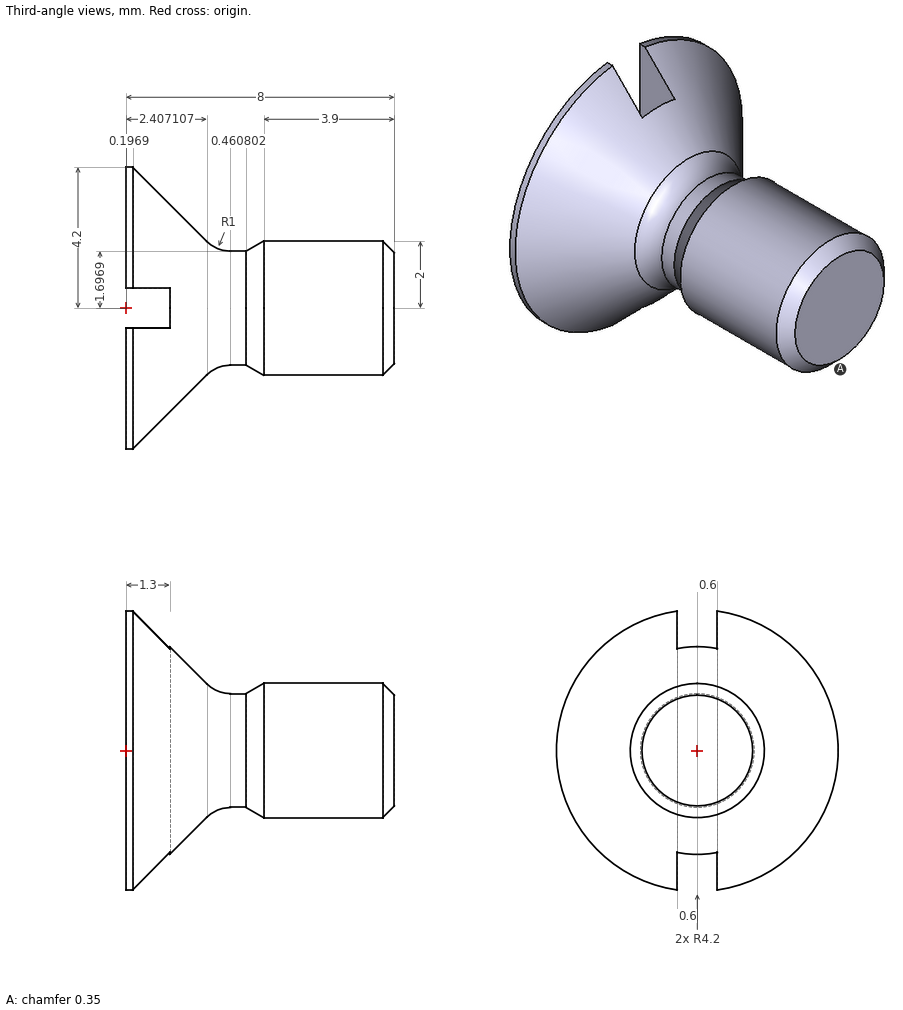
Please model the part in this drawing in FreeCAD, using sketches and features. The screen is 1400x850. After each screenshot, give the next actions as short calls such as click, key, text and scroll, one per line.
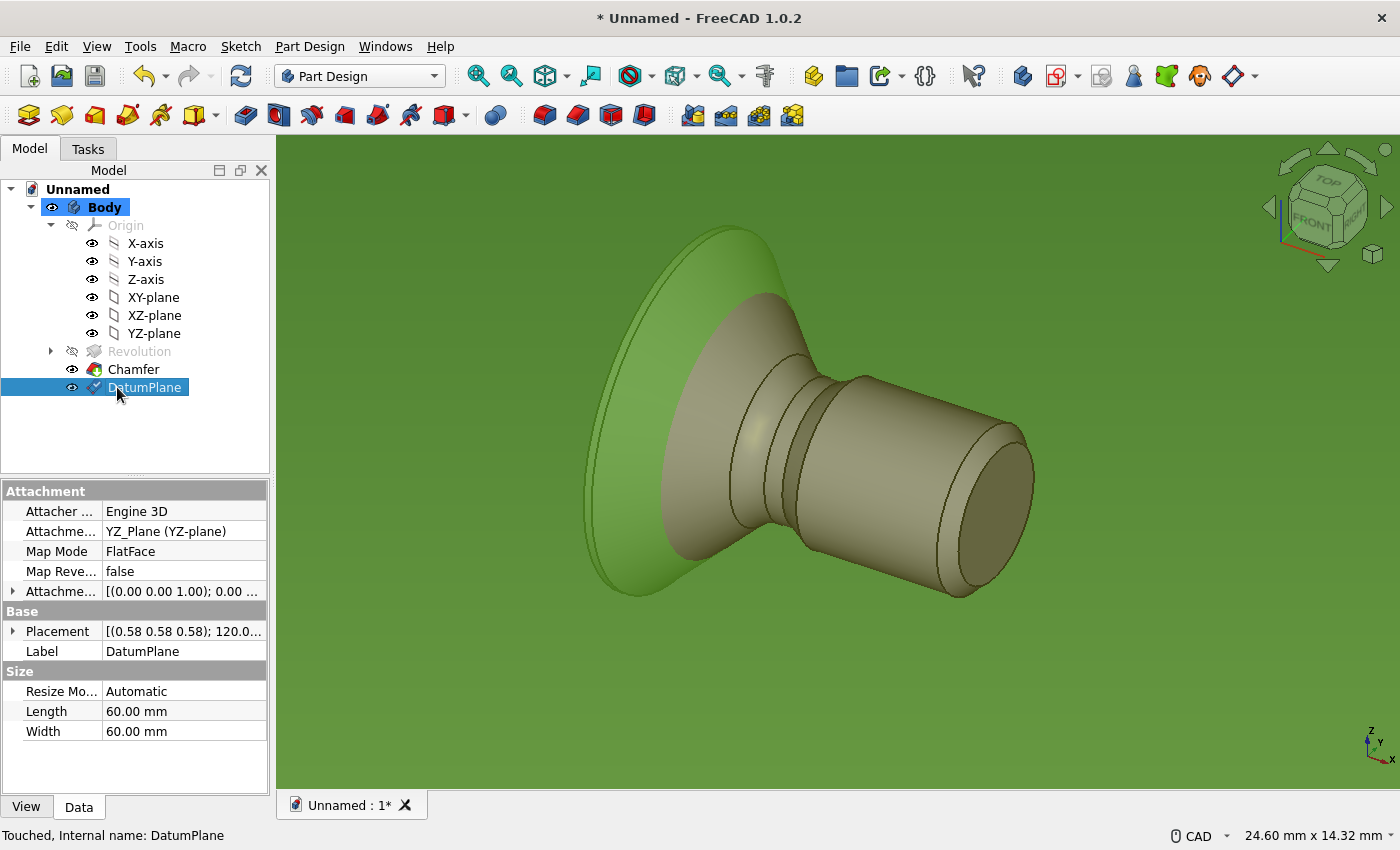
click(1056, 76)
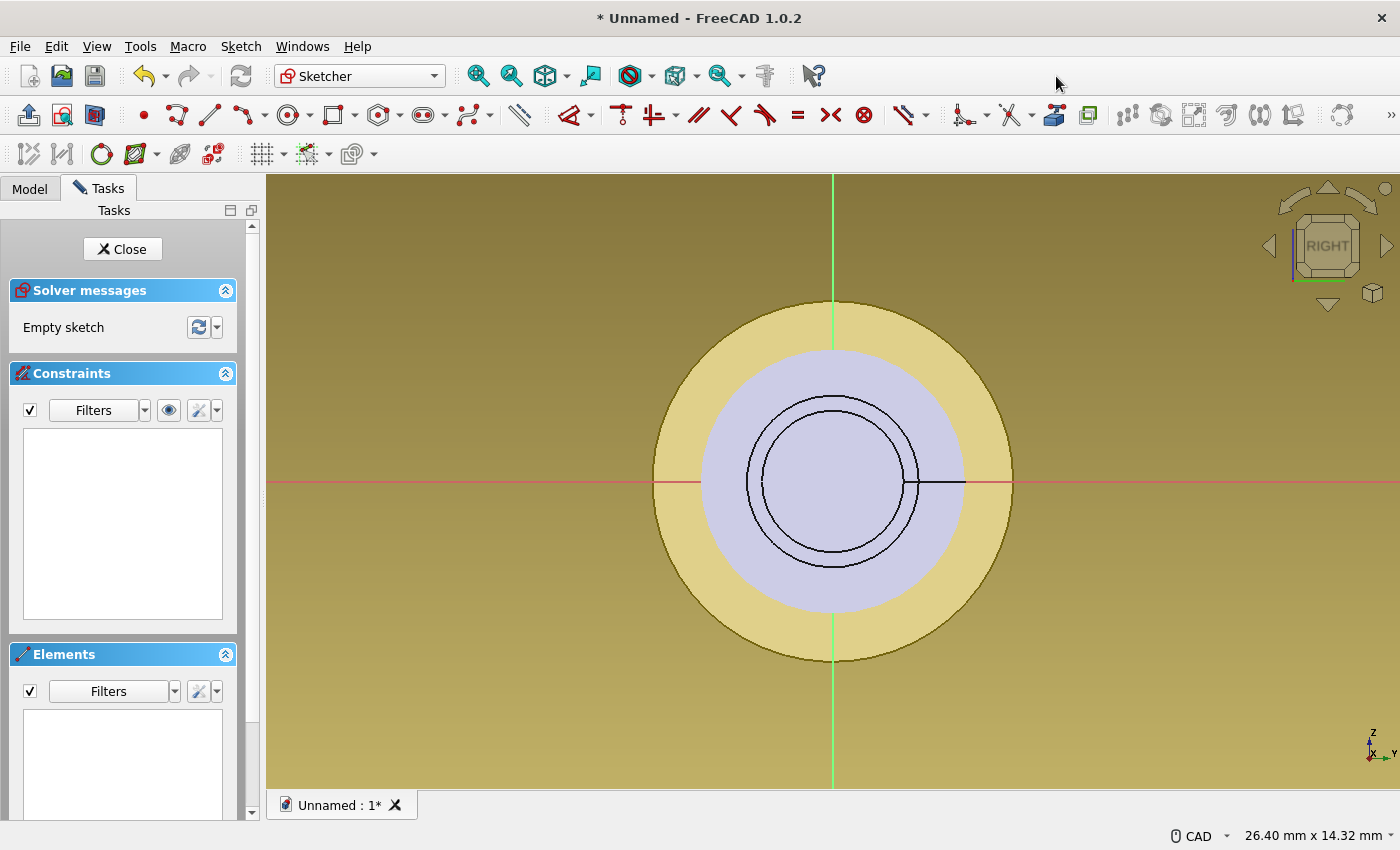
key(q)
key(s)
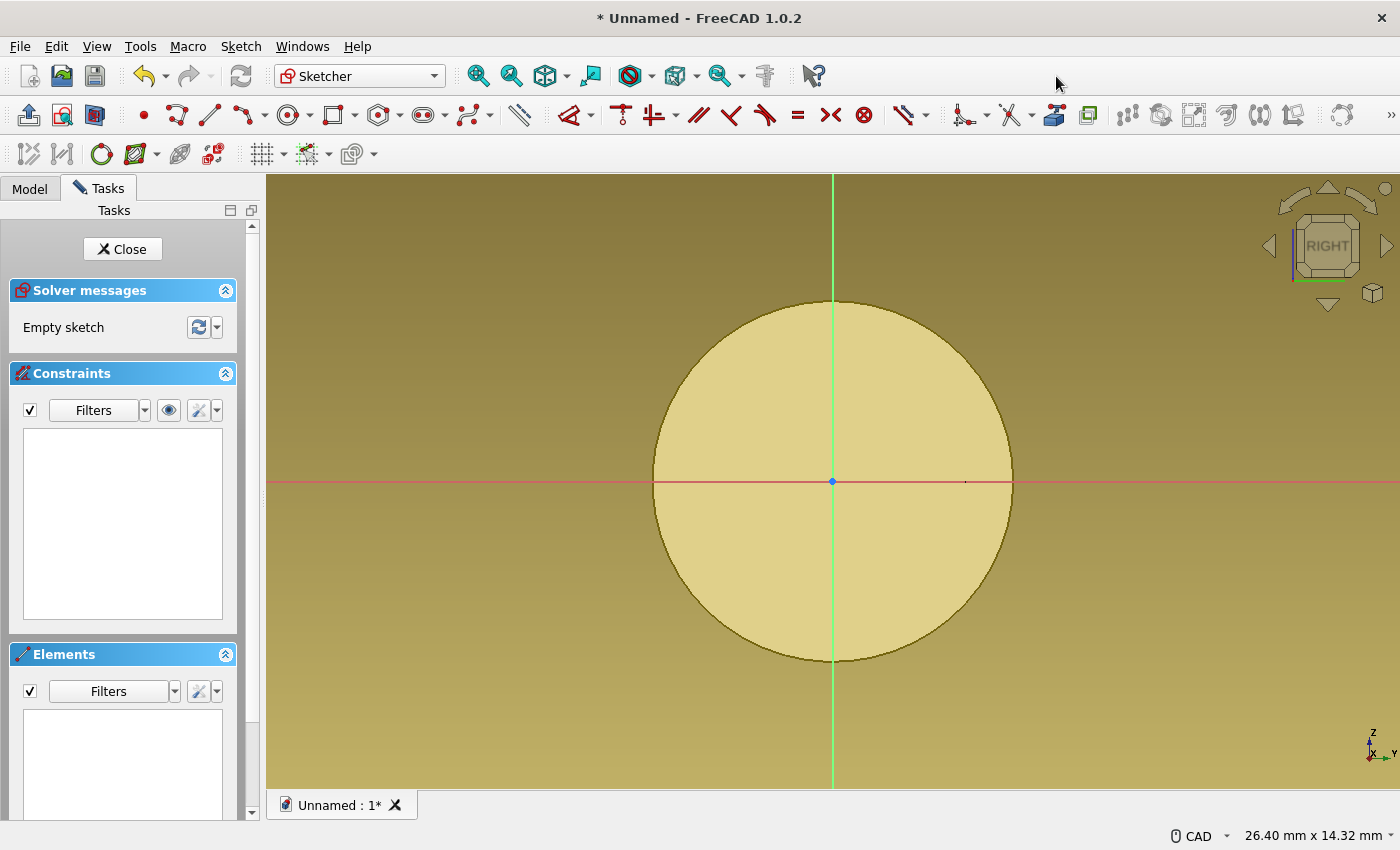
click(210, 116)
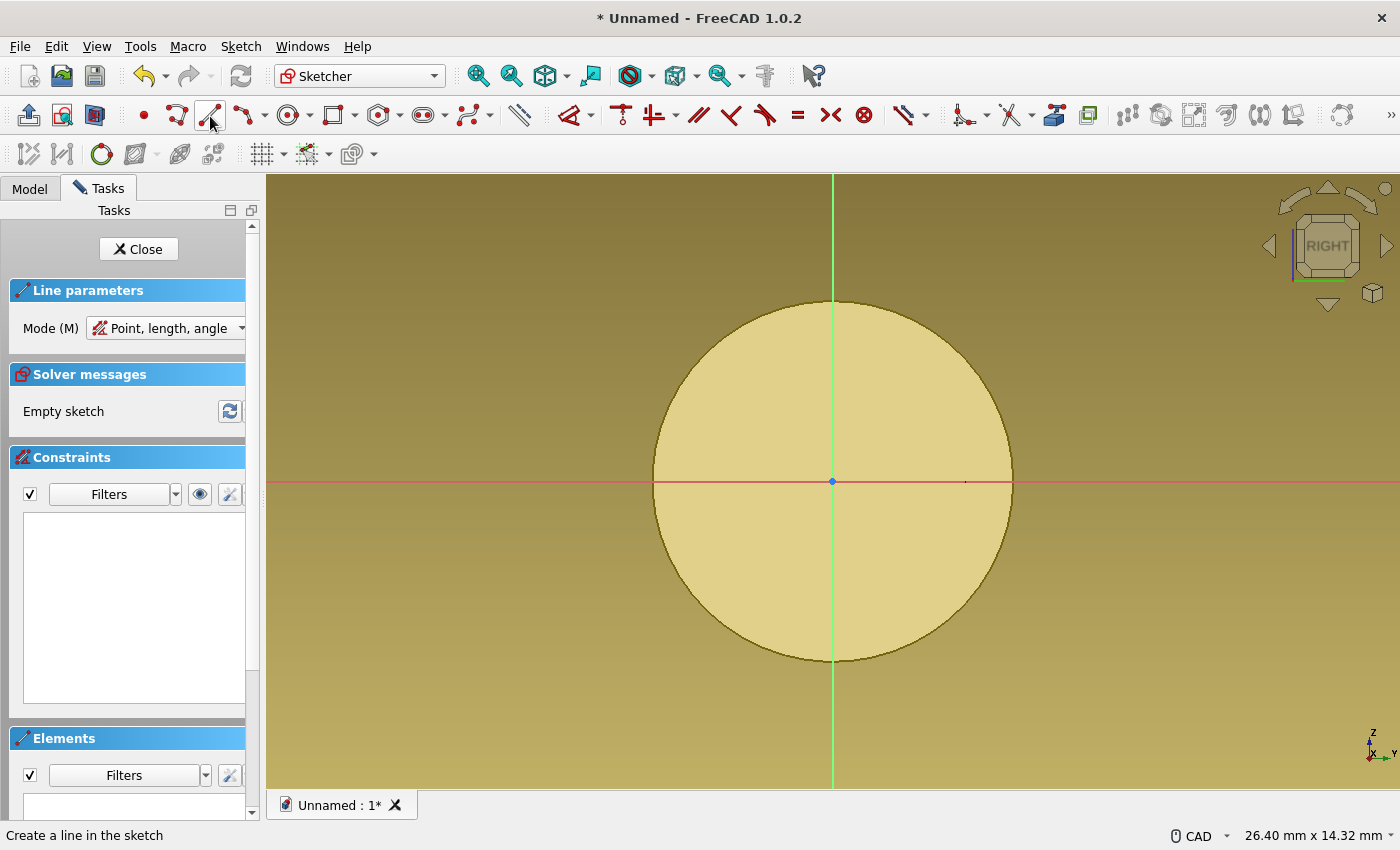
click(859, 303)
click(859, 660)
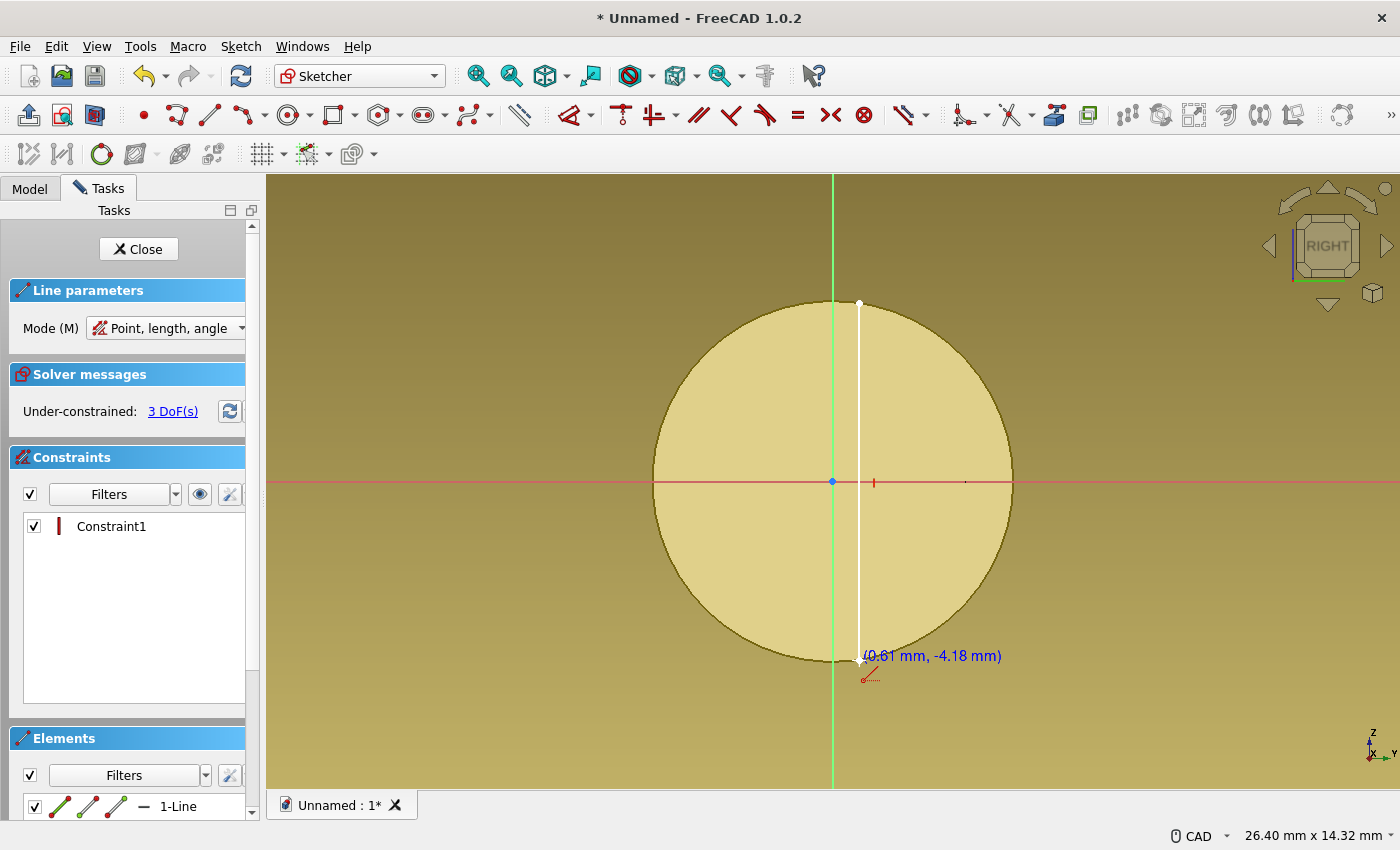
click(807, 660)
click(807, 303)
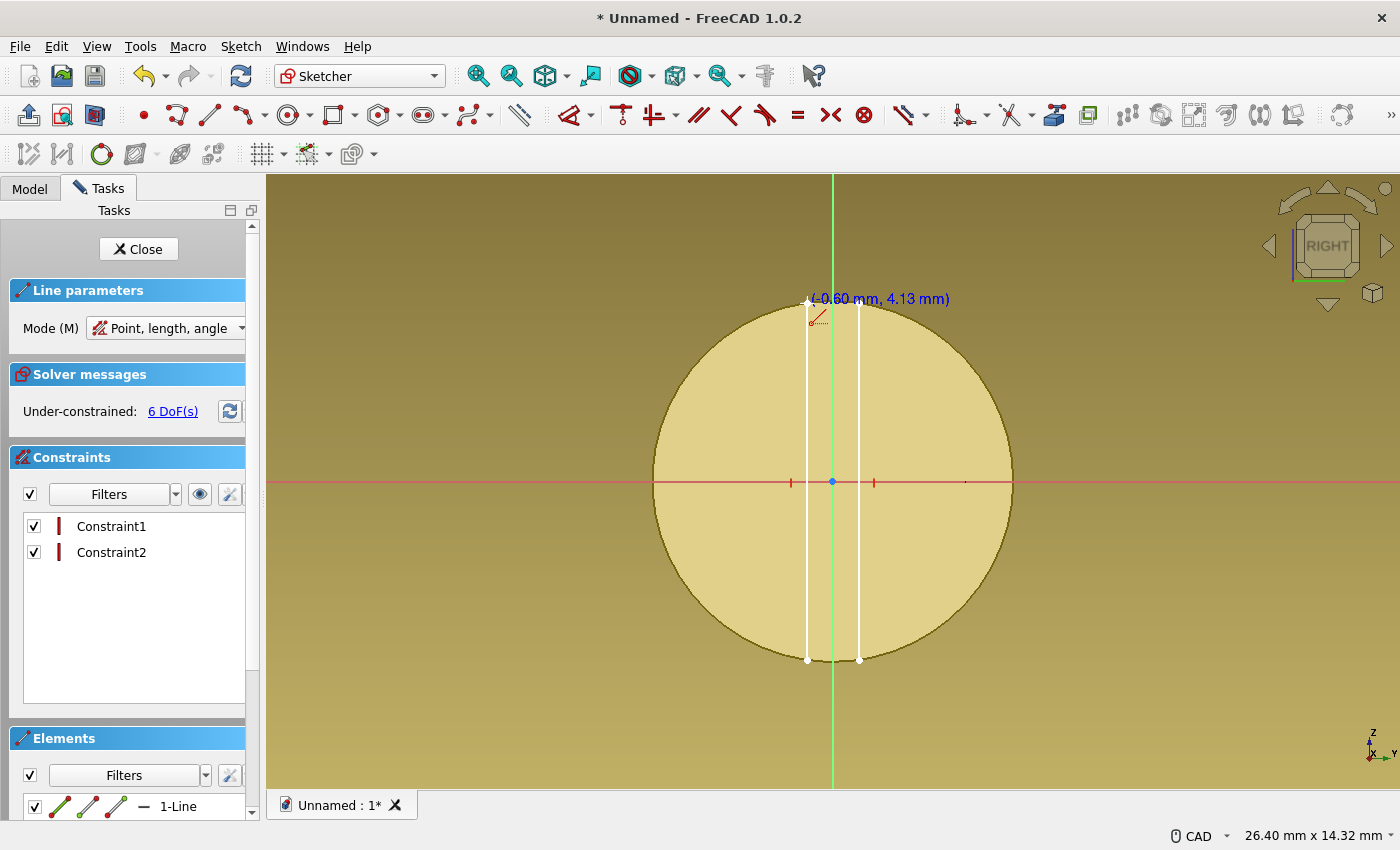
key(g)
key(3)
key(a)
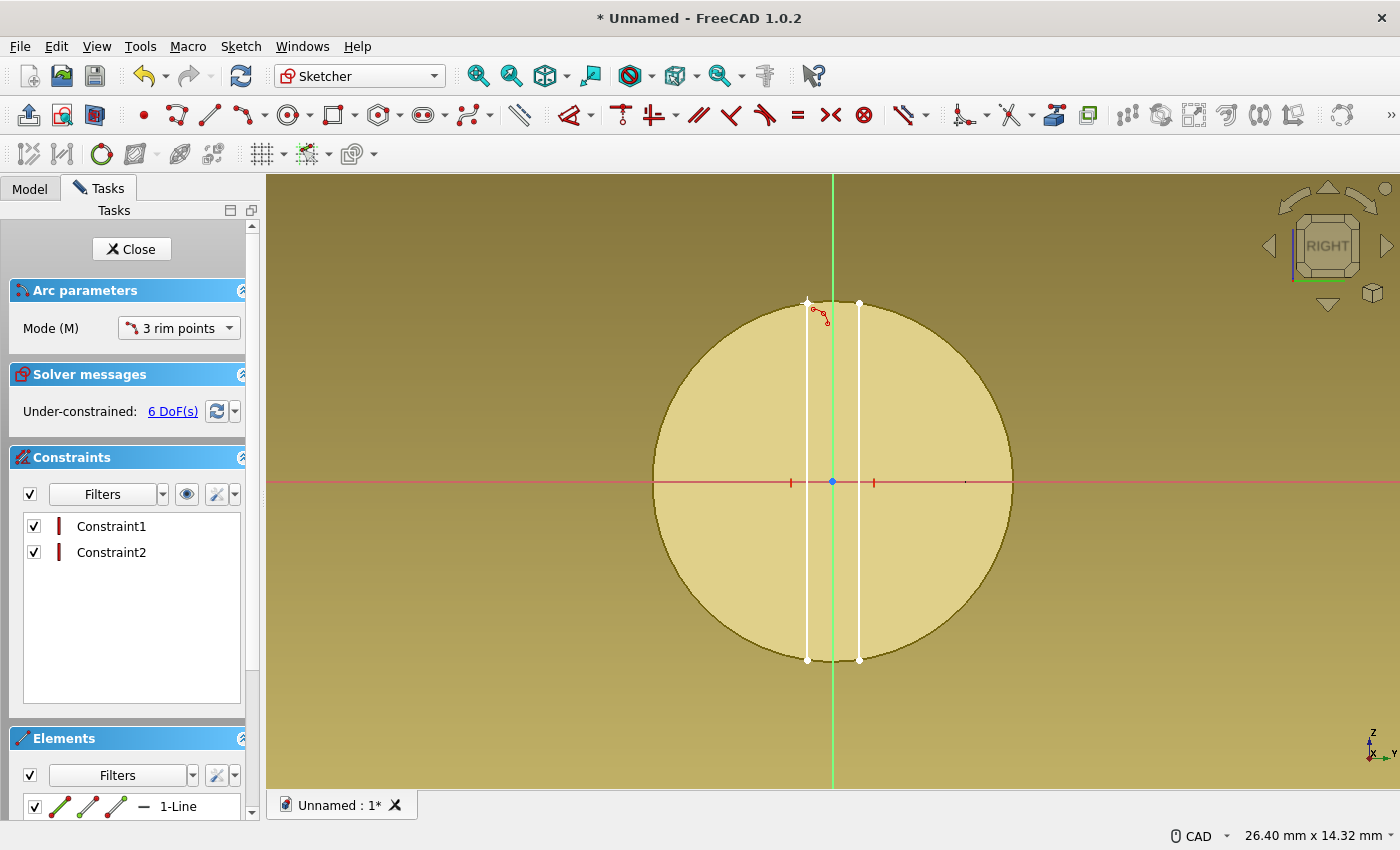
click(859, 661)
click(807, 661)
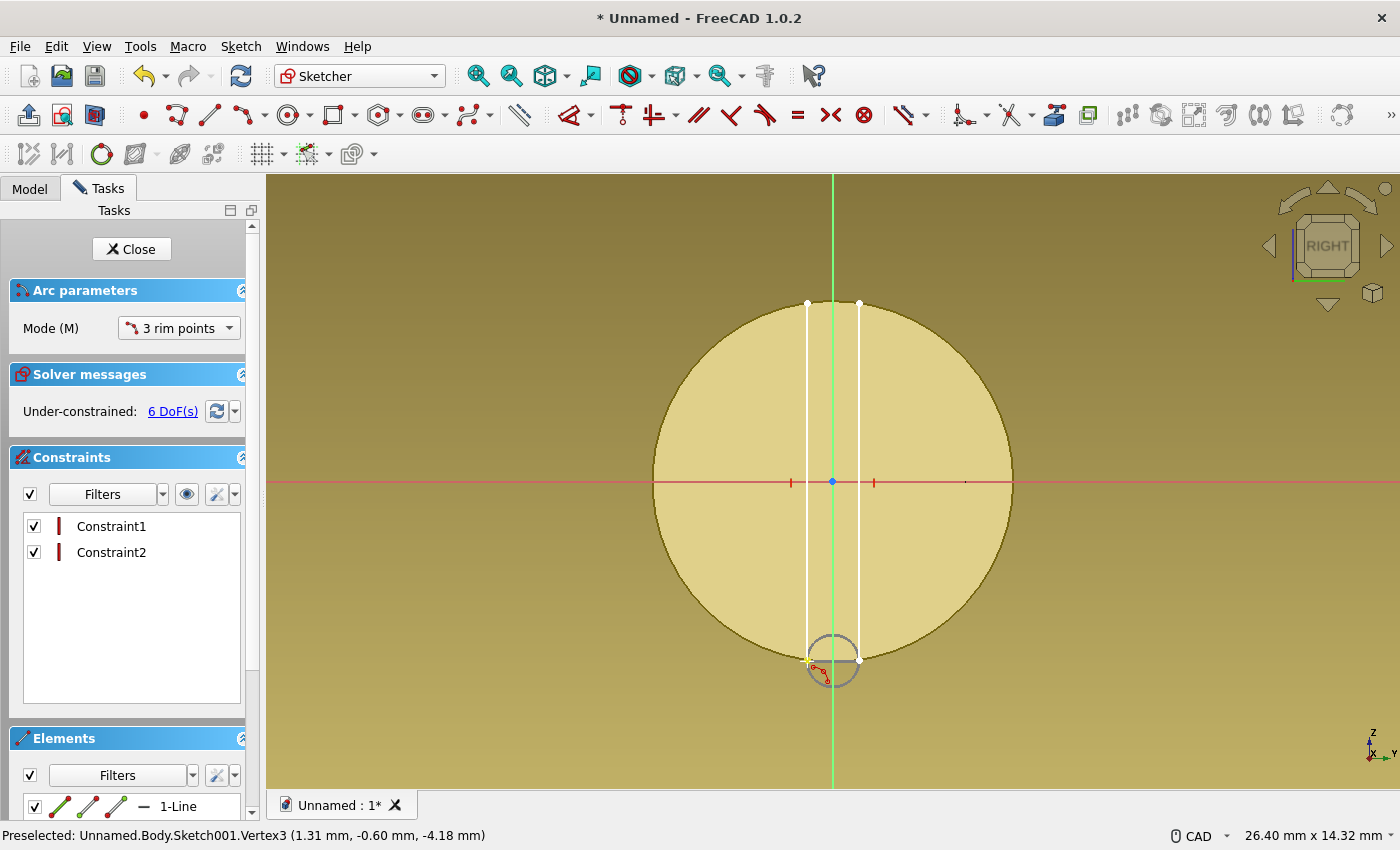
scroll(828, 662, up, 11)